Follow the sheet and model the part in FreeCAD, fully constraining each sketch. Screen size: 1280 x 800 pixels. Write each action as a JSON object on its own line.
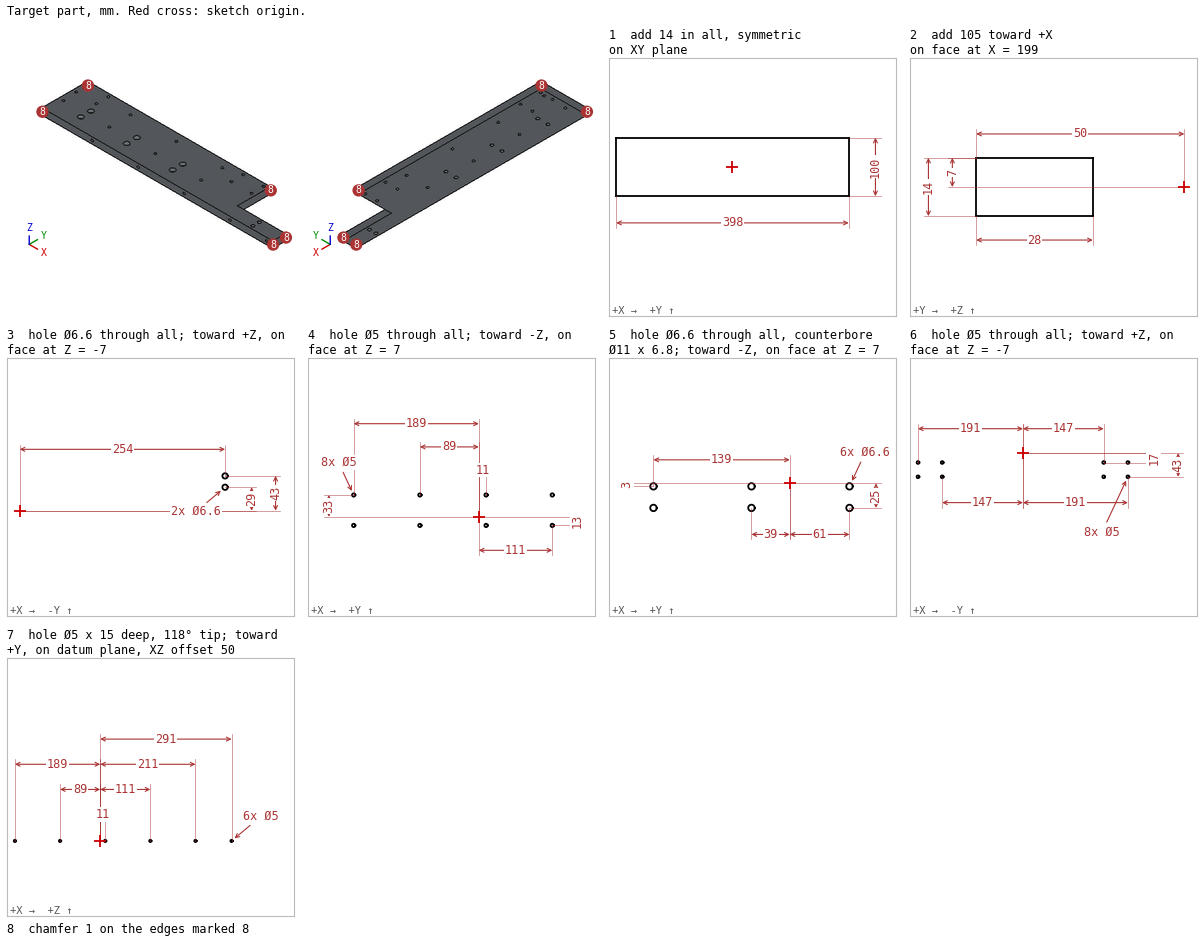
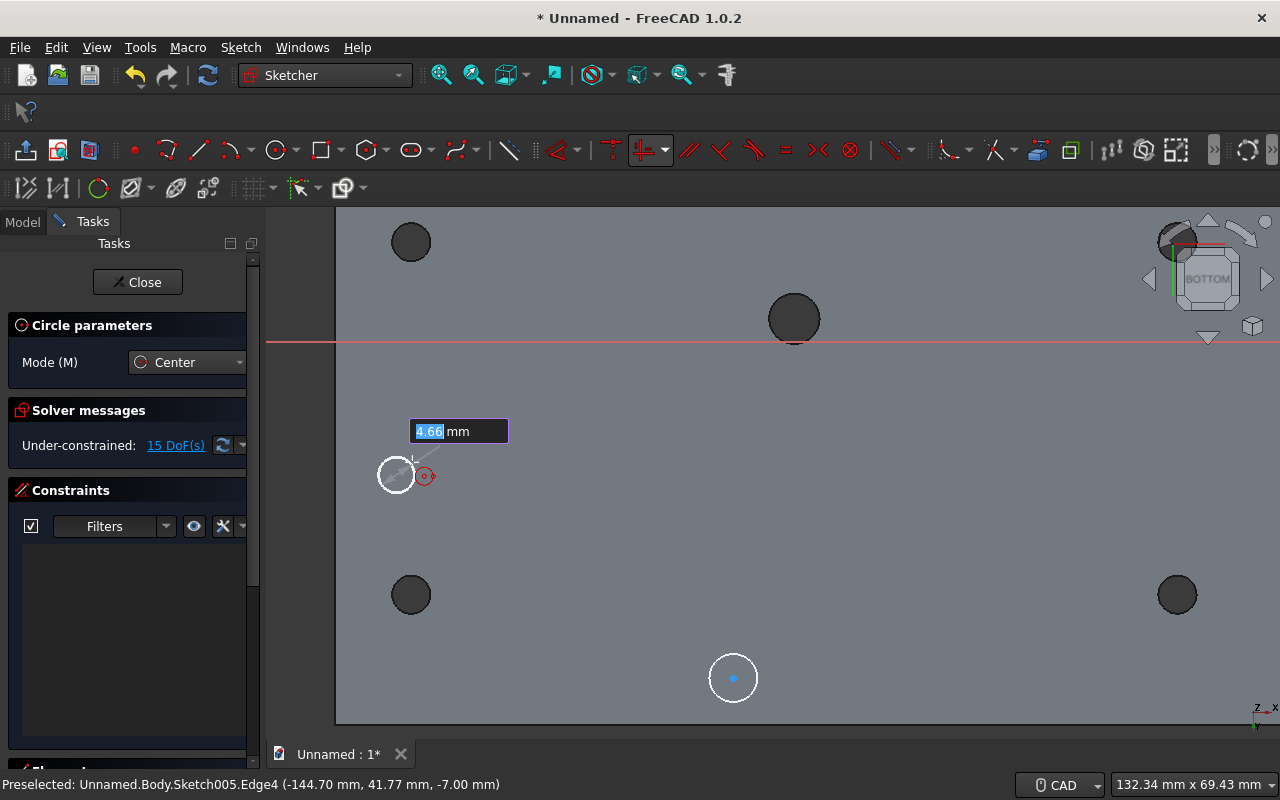
{"action": "left_click", "coordinate": [409, 458]}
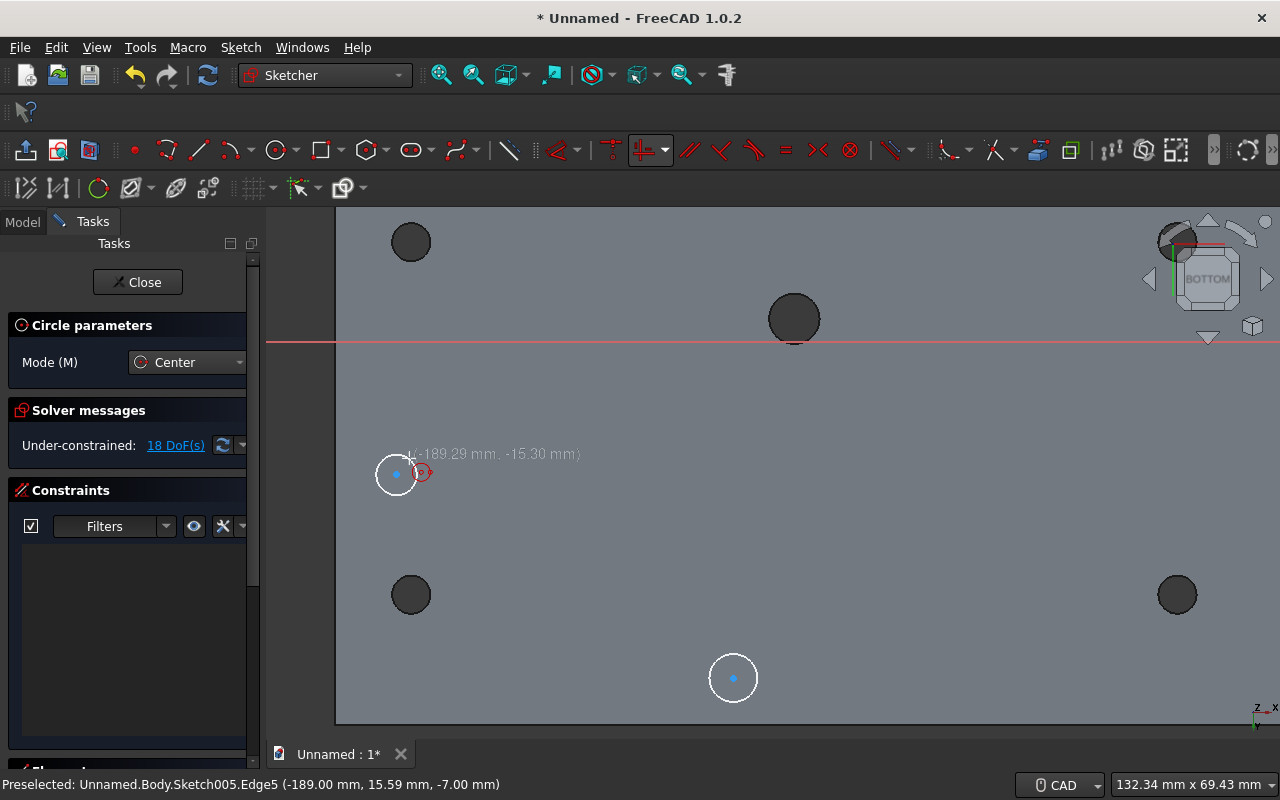
{"action": "scroll", "coordinate": [412, 462], "scroll_direction": "down", "scroll_amount": 8}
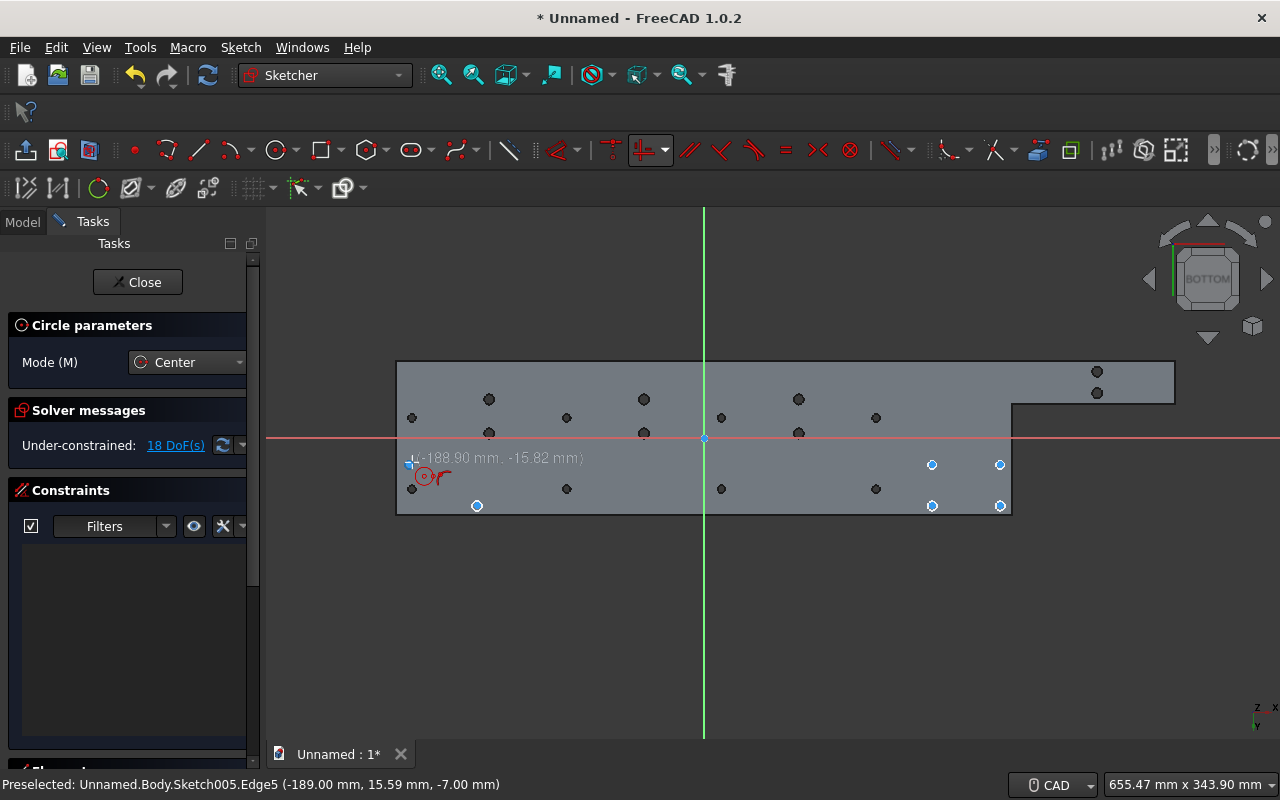
{"action": "left_click", "coordinate": [477, 464]}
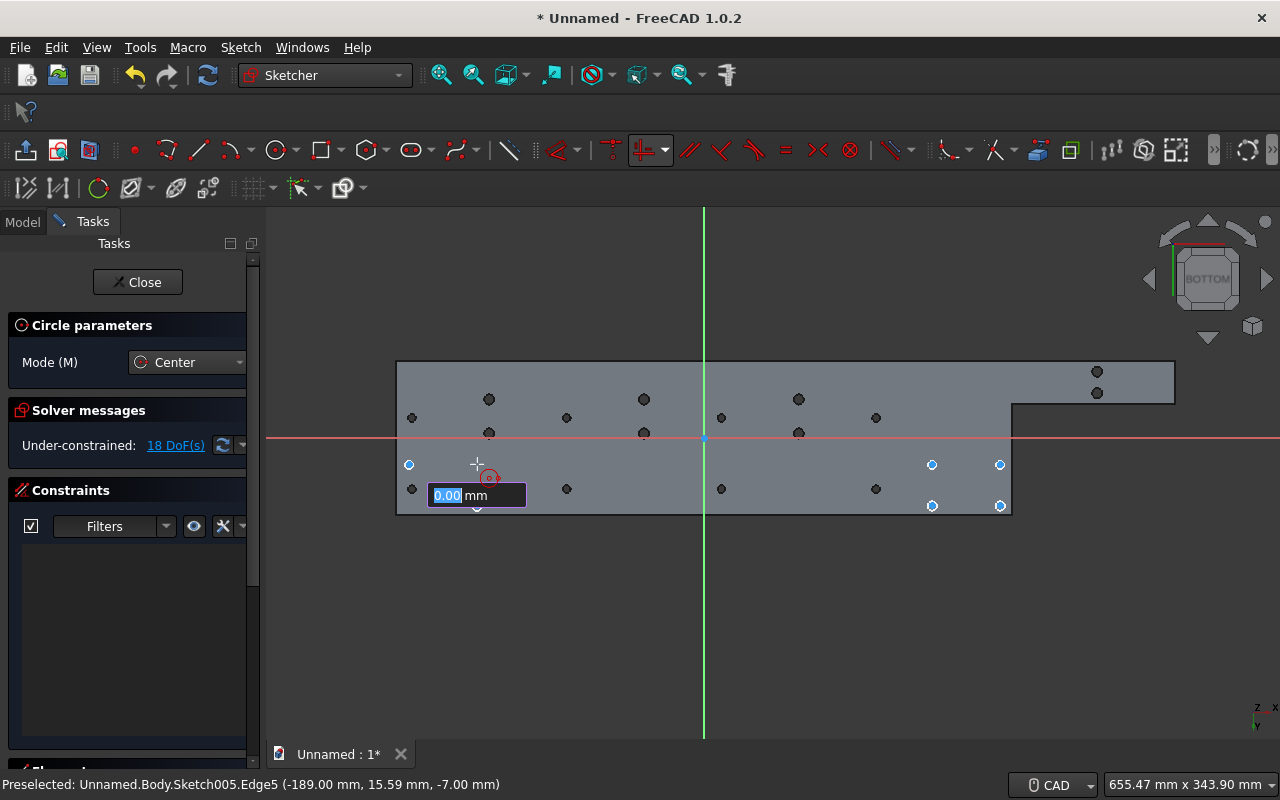
{"action": "scroll", "coordinate": [480, 462], "scroll_direction": "up", "scroll_amount": 8}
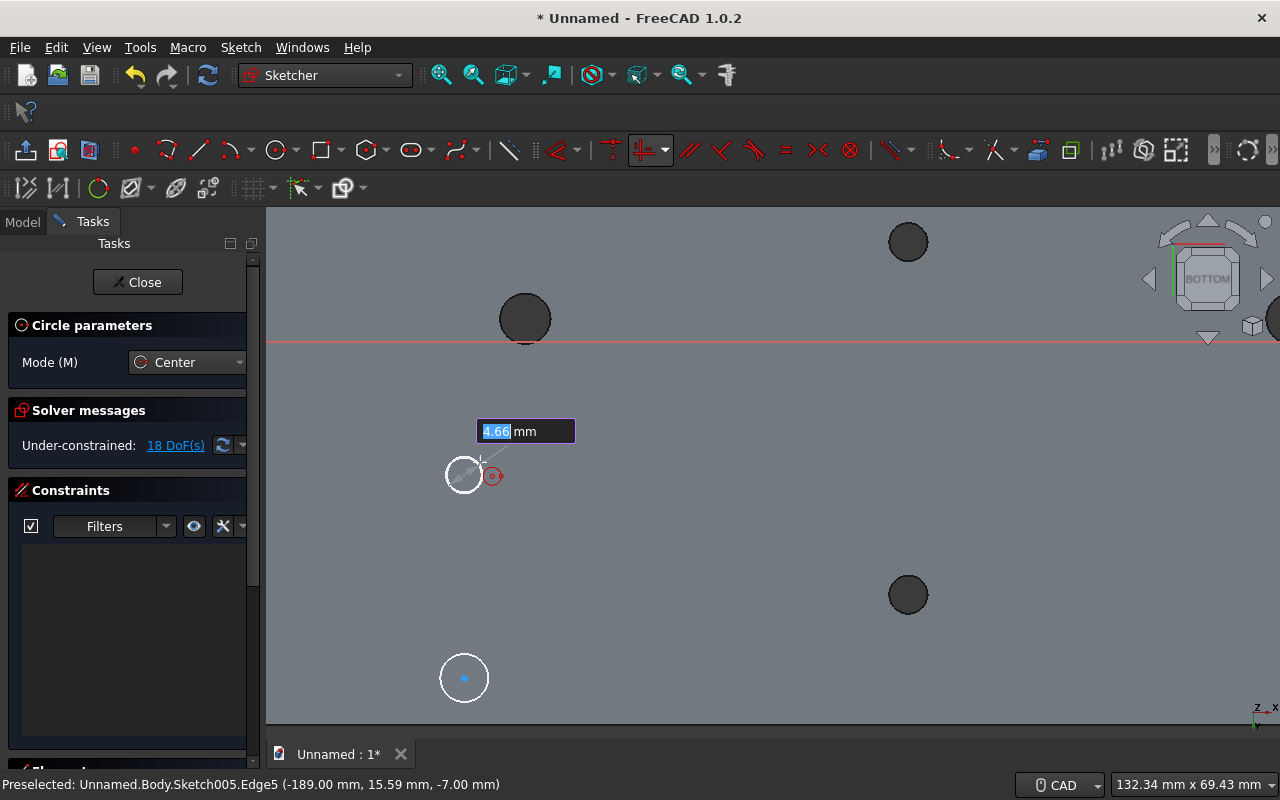
{"action": "left_click", "coordinate": [478, 458]}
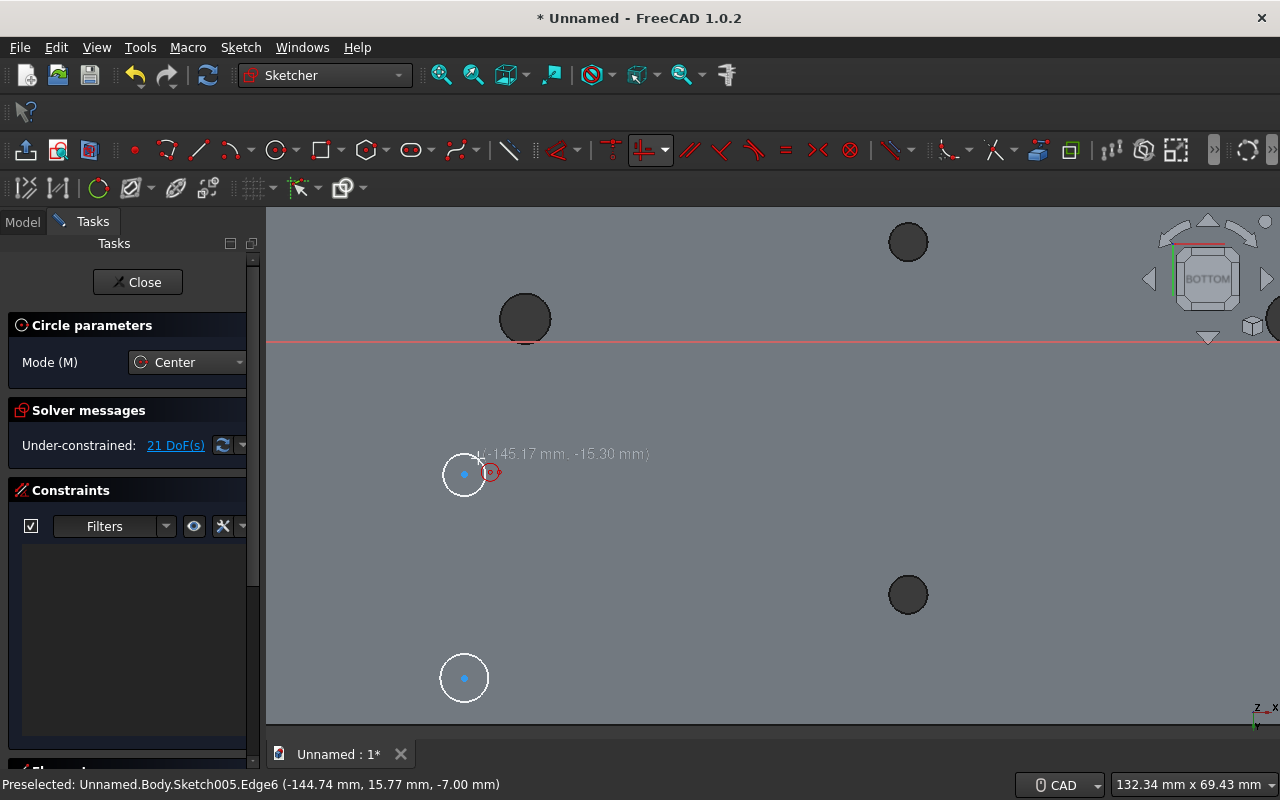
{"action": "scroll", "coordinate": [480, 462], "scroll_direction": "down", "scroll_amount": 8}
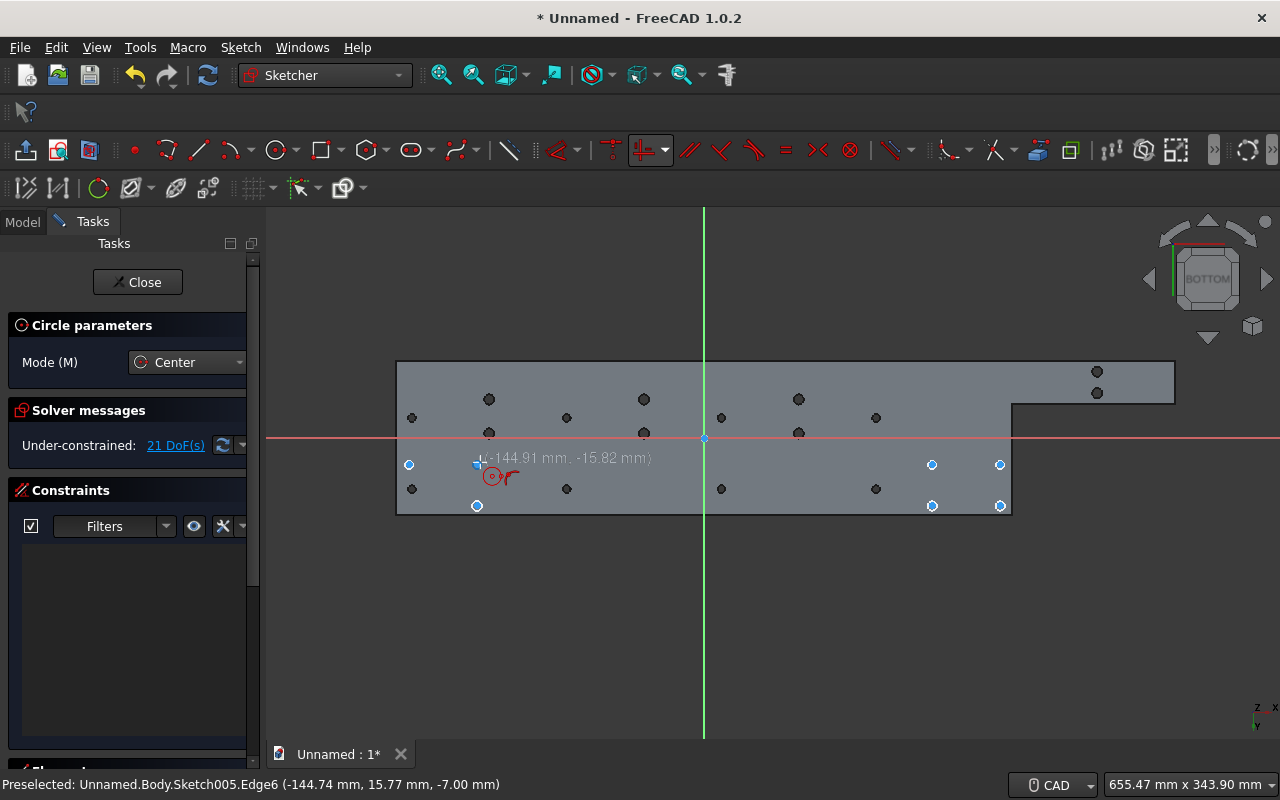
{"action": "scroll", "coordinate": [409, 505], "scroll_direction": "up", "scroll_amount": 9}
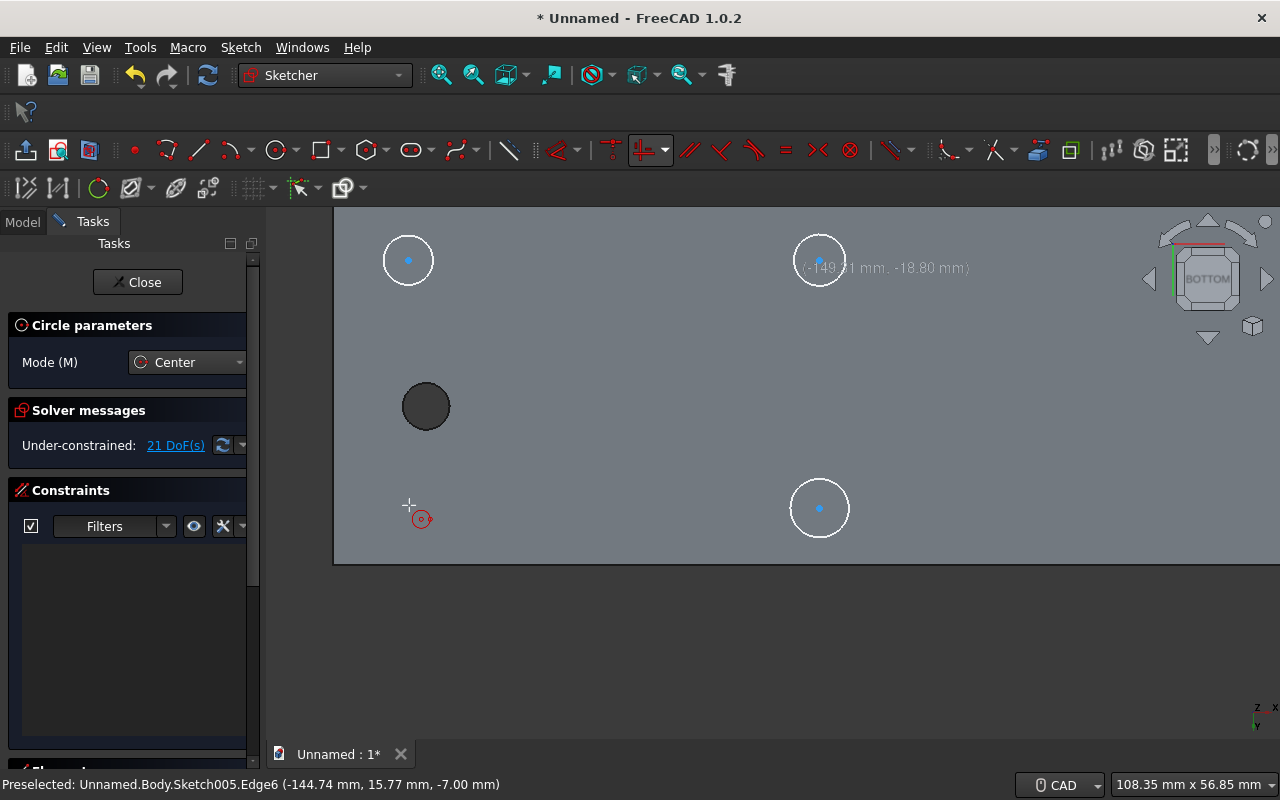
{"action": "scroll", "coordinate": [409, 505], "scroll_direction": "down", "scroll_amount": 9}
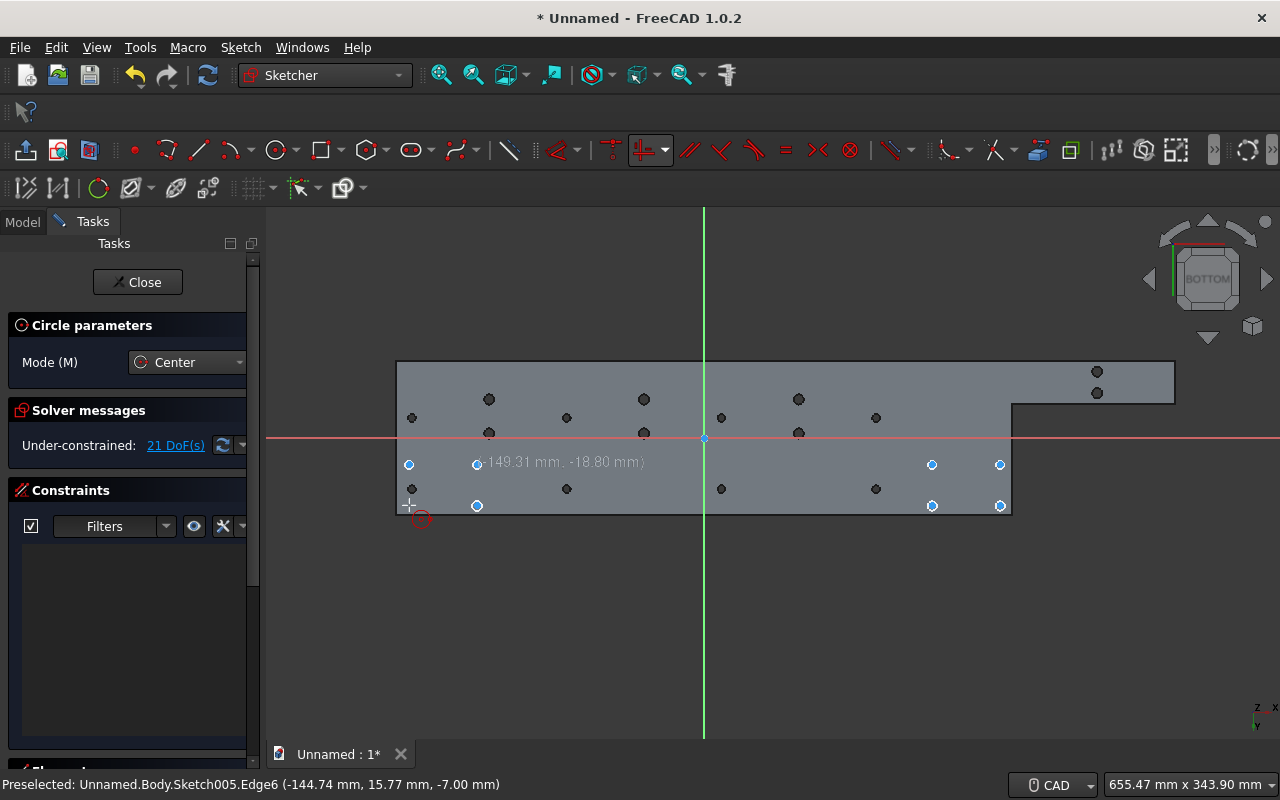
{"action": "left_click", "coordinate": [409, 505]}